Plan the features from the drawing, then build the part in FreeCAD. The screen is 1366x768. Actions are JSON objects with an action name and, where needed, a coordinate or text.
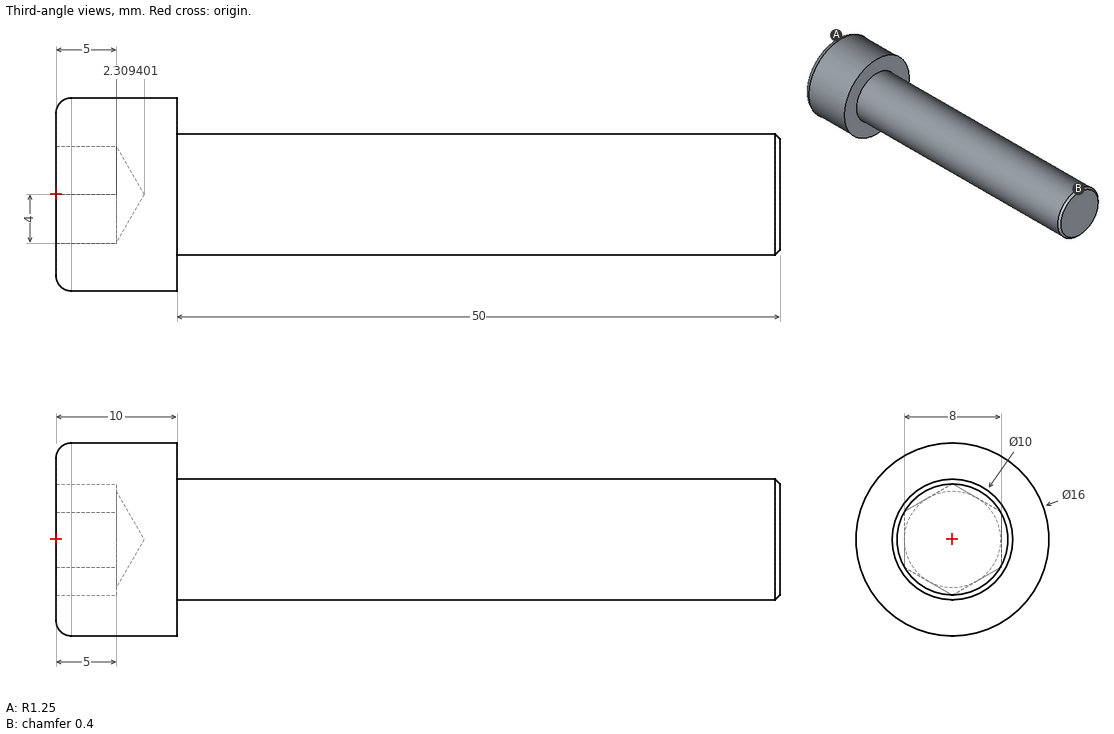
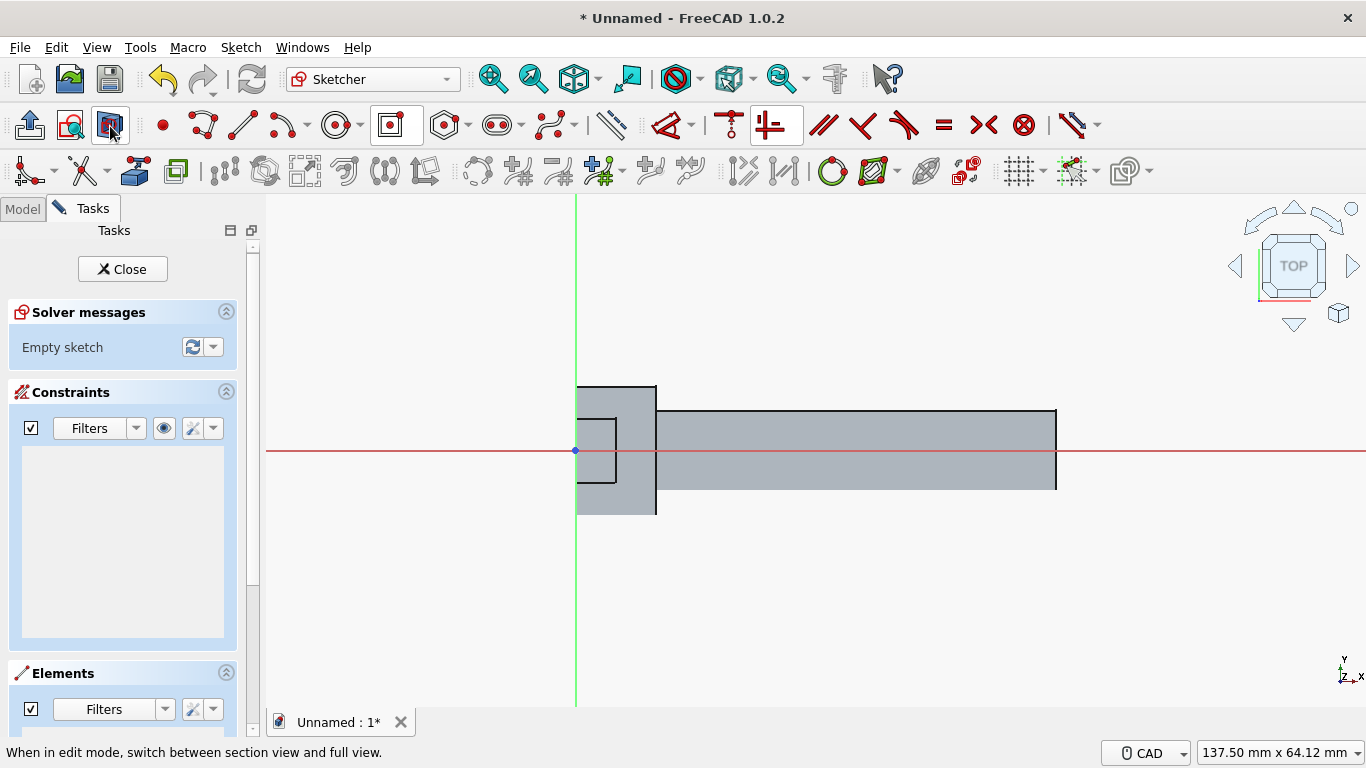
{"action": "scroll", "coordinate": [591, 468], "scroll_direction": "up", "scroll_amount": 12}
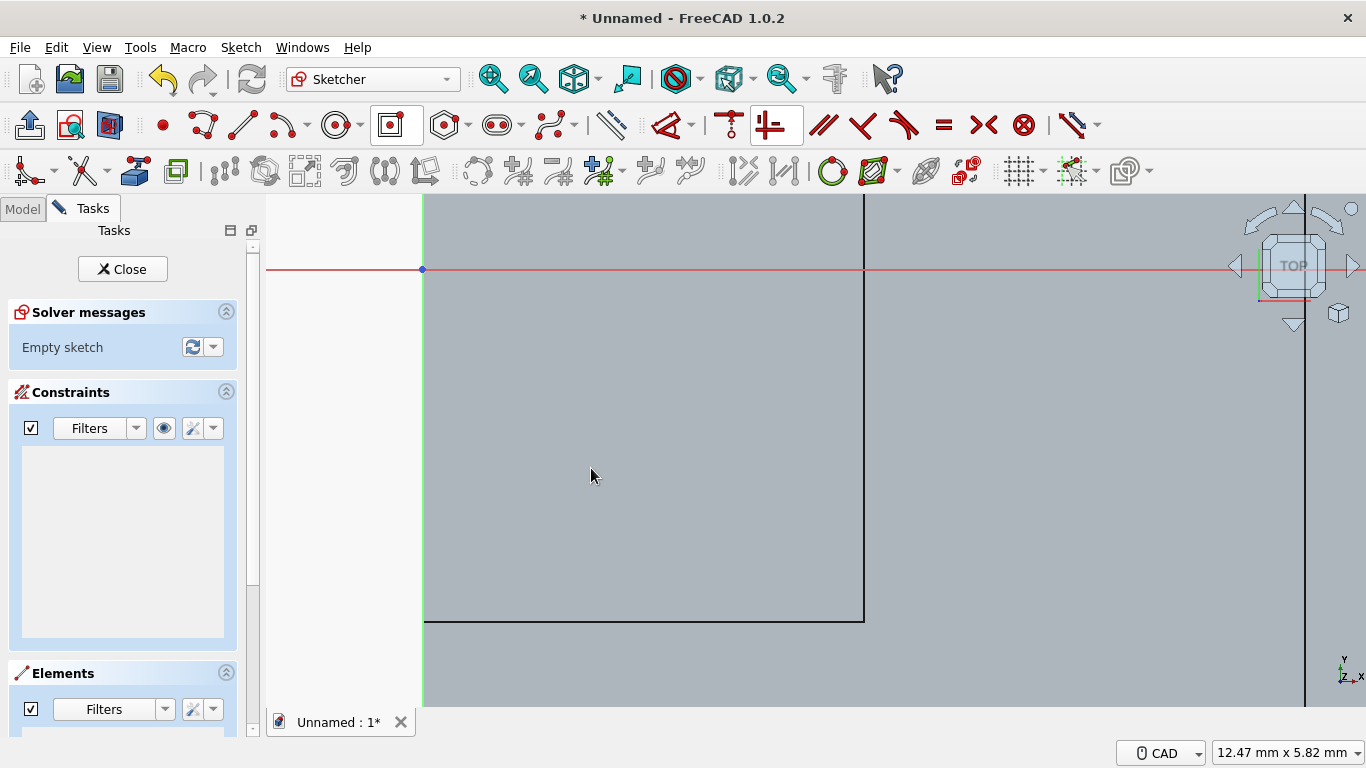
{"action": "left_click", "coordinate": [204, 126]}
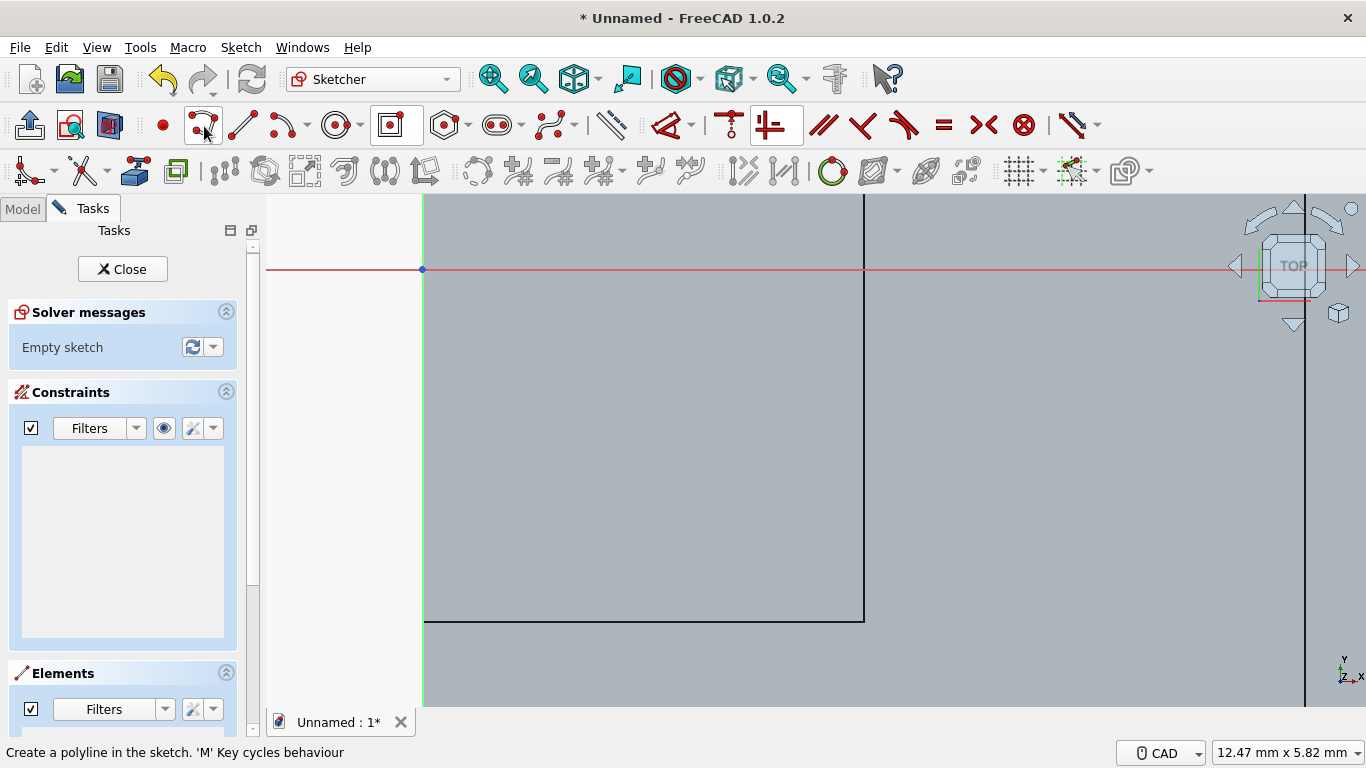
{"action": "left_click", "coordinate": [864, 270]}
{"action": "left_click", "coordinate": [864, 622]}
{"action": "left_click", "coordinate": [1067, 279]}
{"action": "left_click", "coordinate": [864, 270]}
{"action": "key", "text": "Escape"}
{"action": "key", "text": "Escape"}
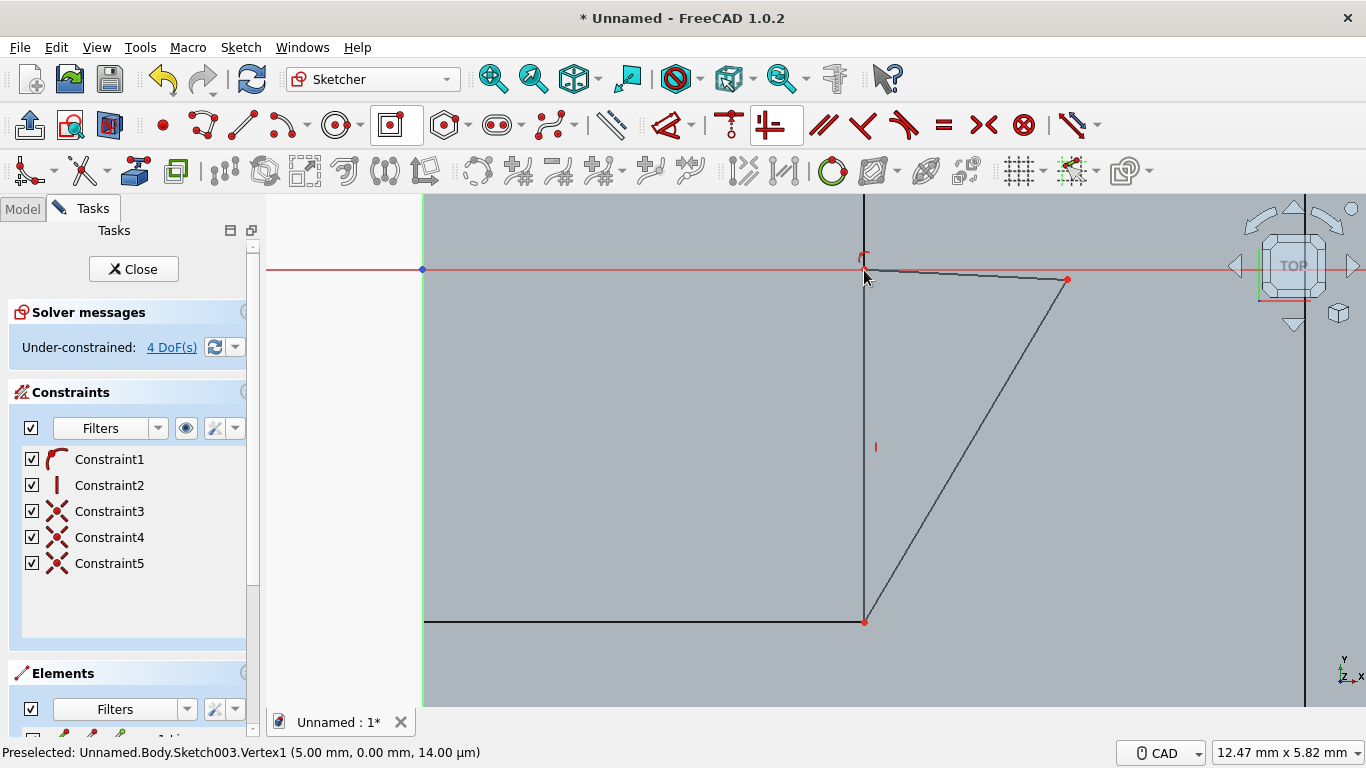
{"action": "left_click", "coordinate": [925, 273]}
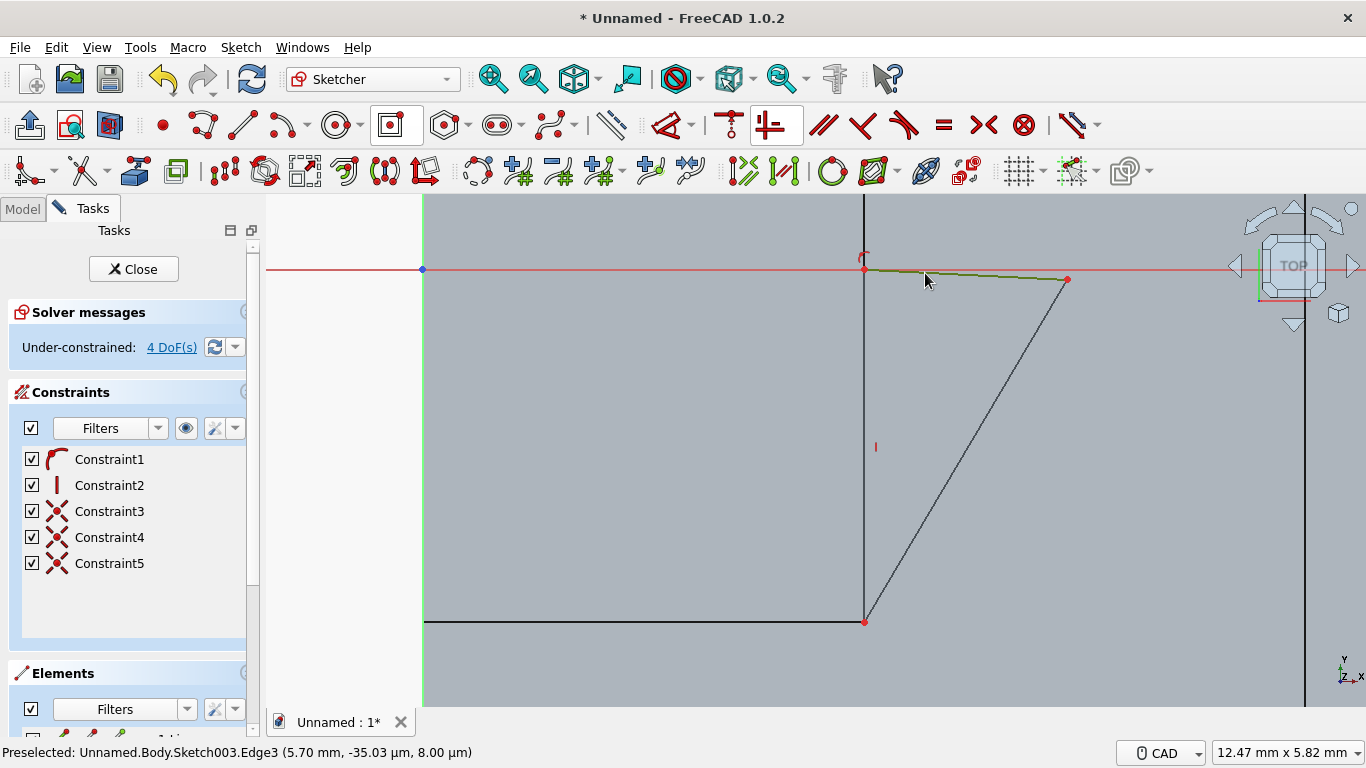
{"action": "key", "text": "h"}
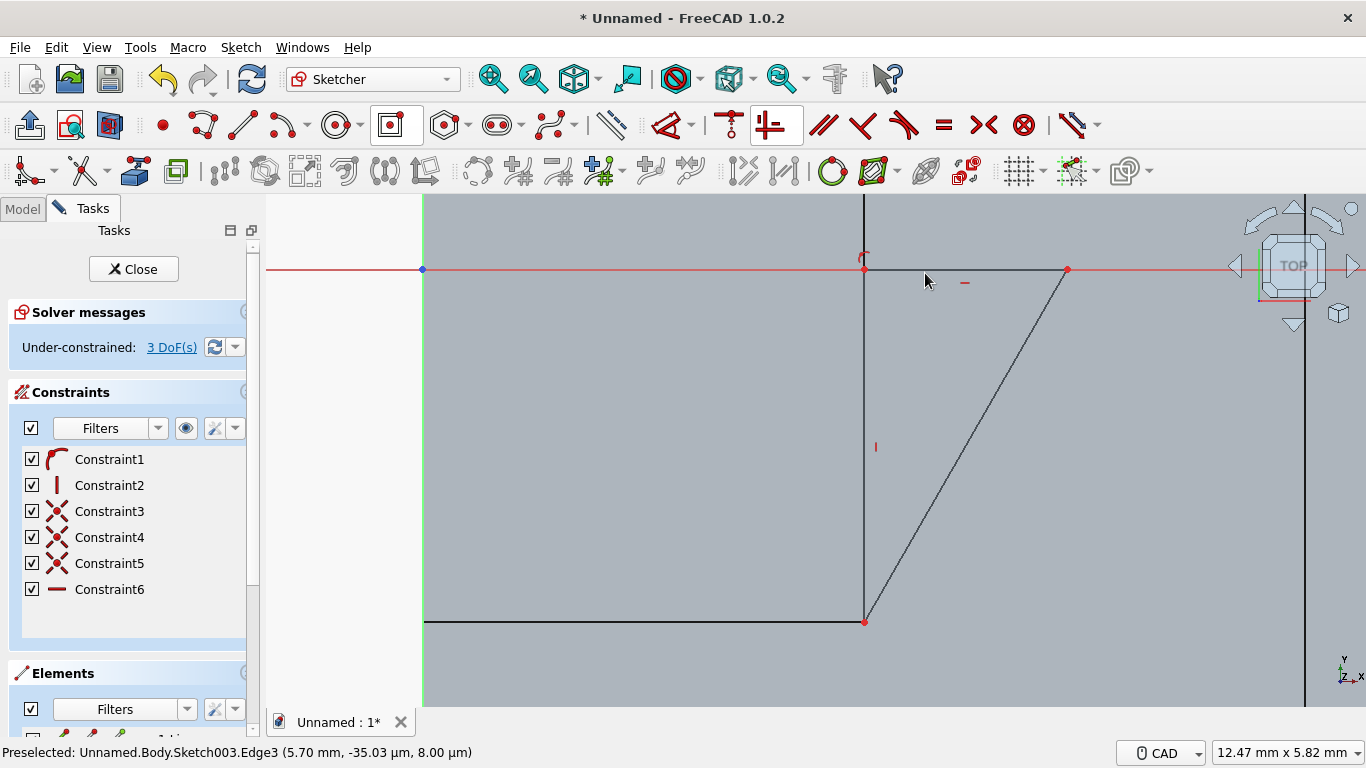
{"action": "key", "text": "d"}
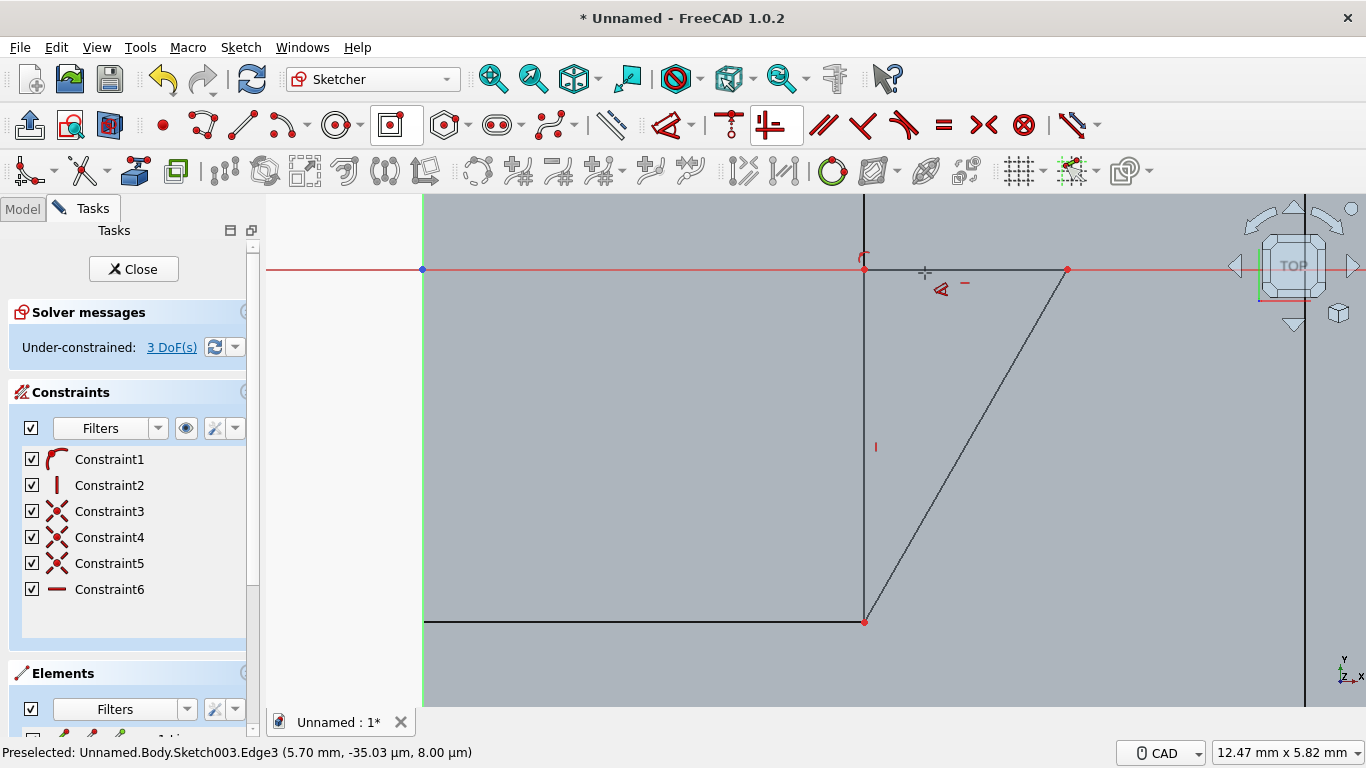
{"action": "left_click", "coordinate": [864, 376]}
{"action": "left_click", "coordinate": [898, 446]}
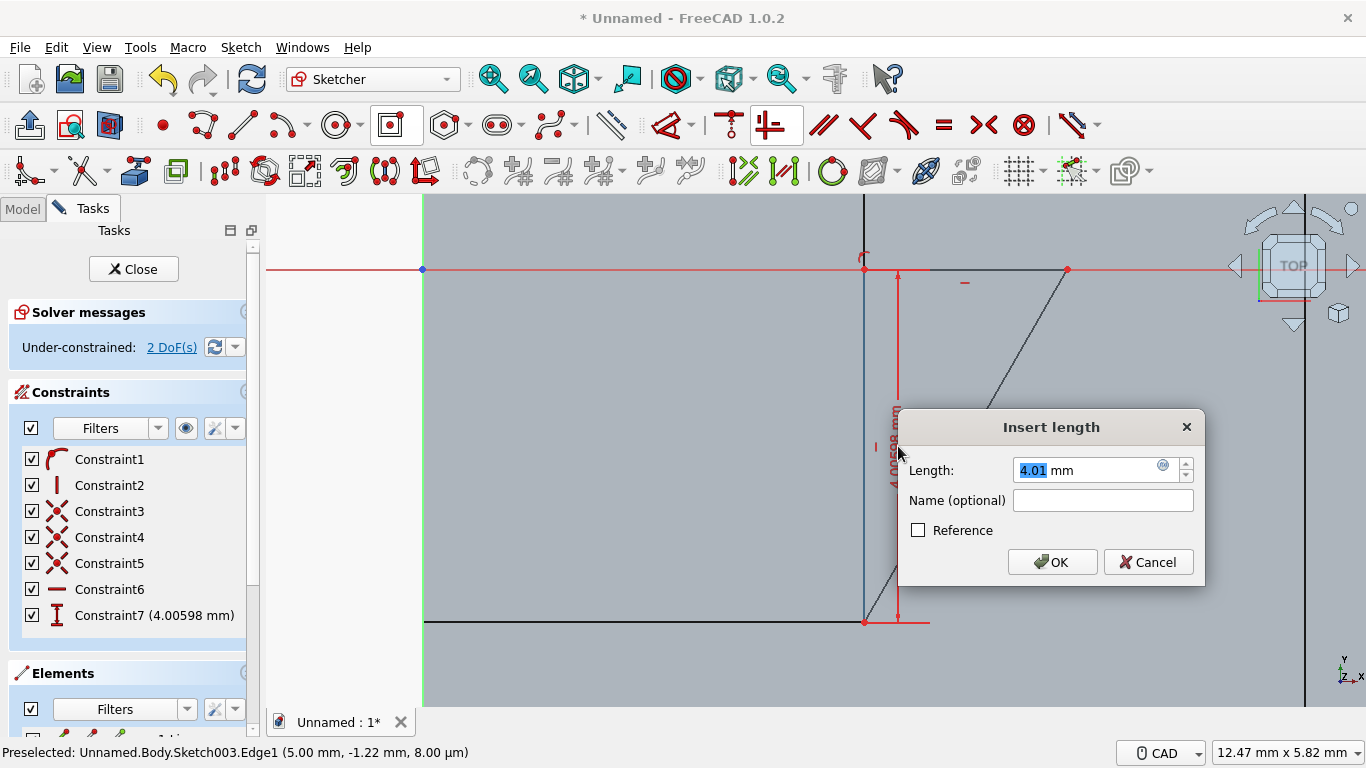
{"action": "type", "text": "4"}
{"action": "key", "text": "Return"}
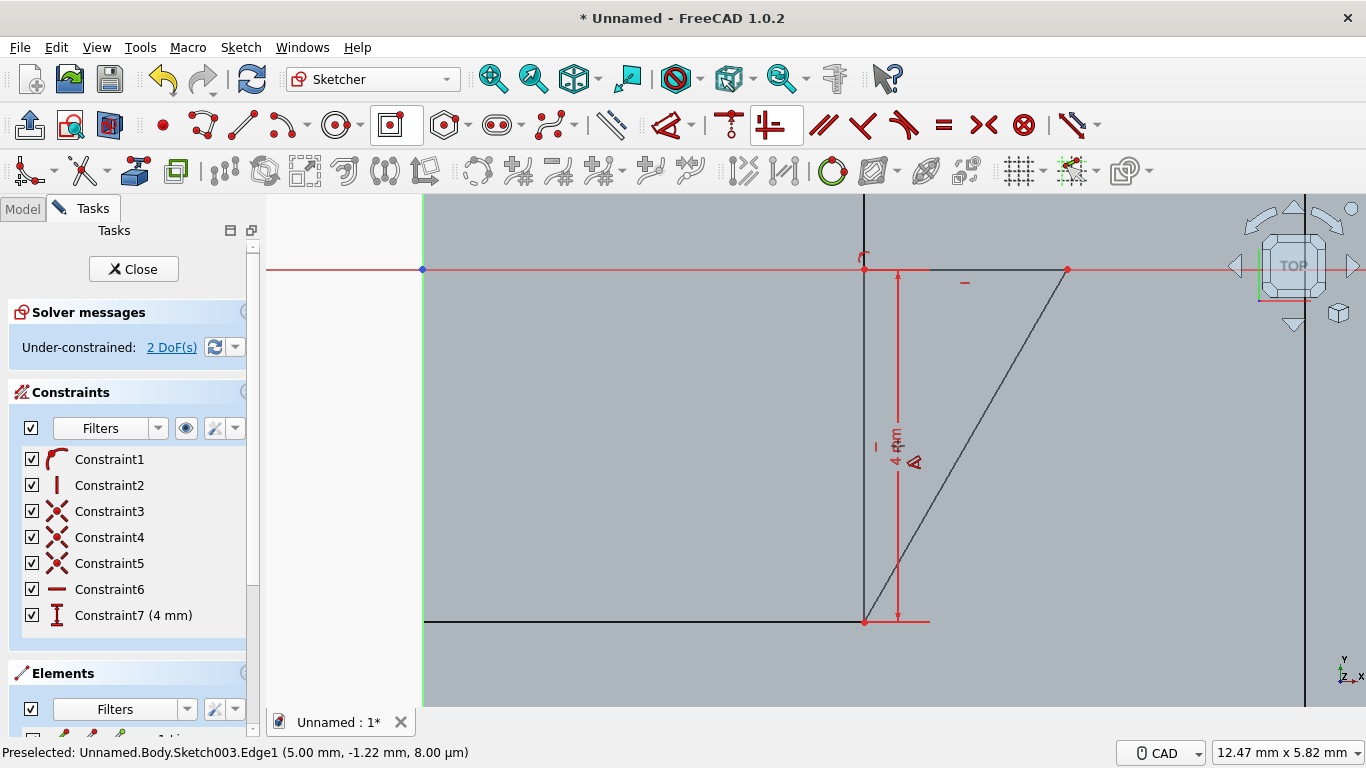
{"action": "left_click", "coordinate": [864, 270]}
{"action": "left_click", "coordinate": [643, 236]}